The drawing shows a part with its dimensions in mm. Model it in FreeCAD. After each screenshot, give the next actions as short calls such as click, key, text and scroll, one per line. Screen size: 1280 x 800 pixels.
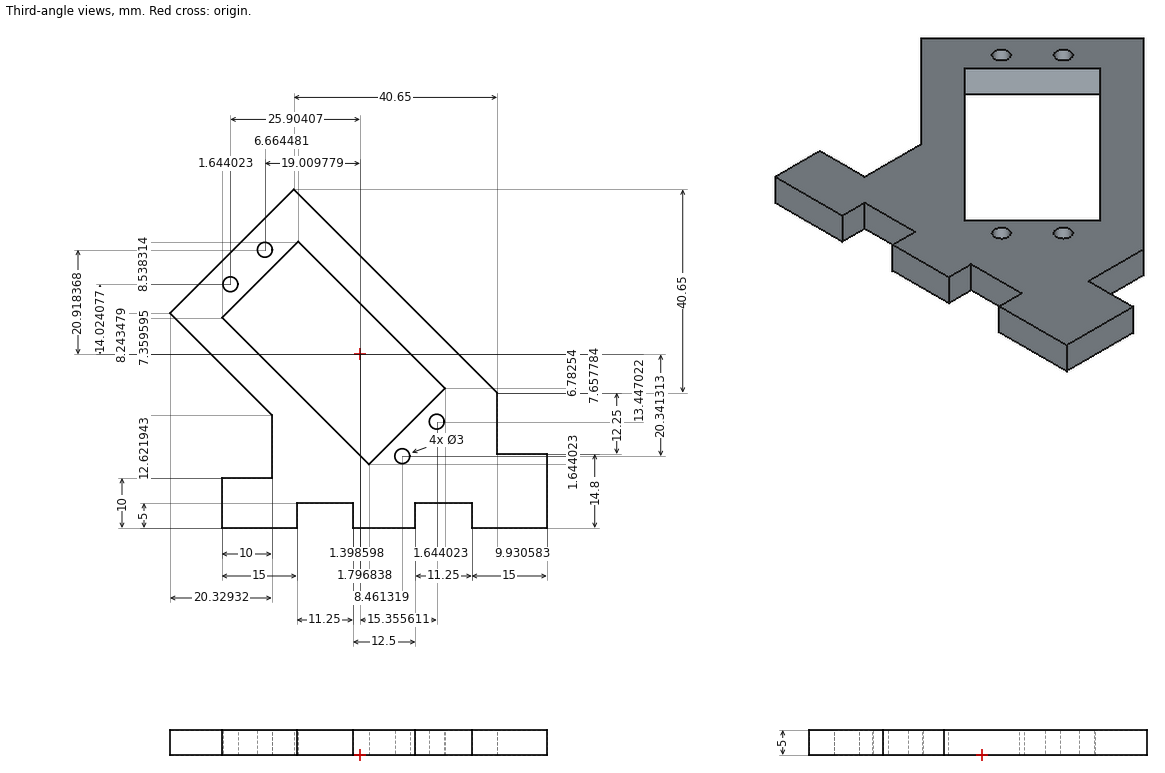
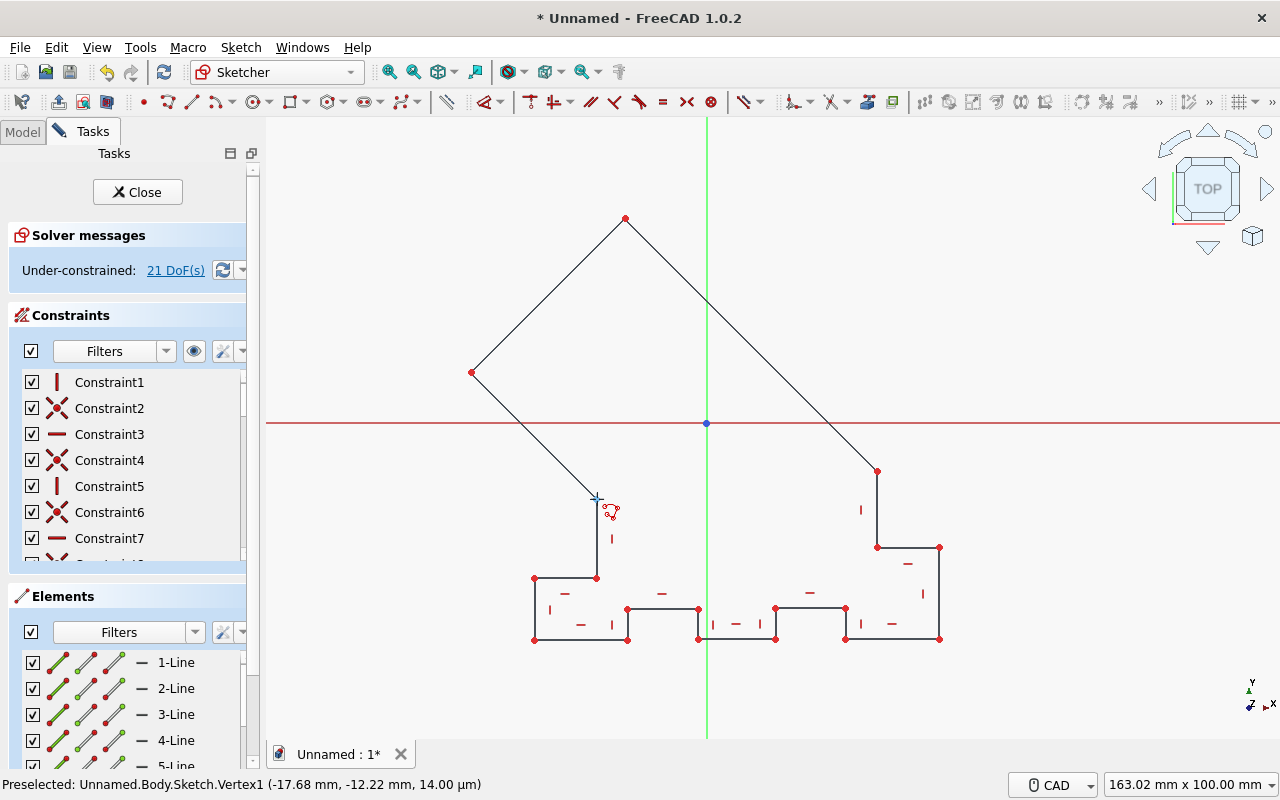
click(813, 465)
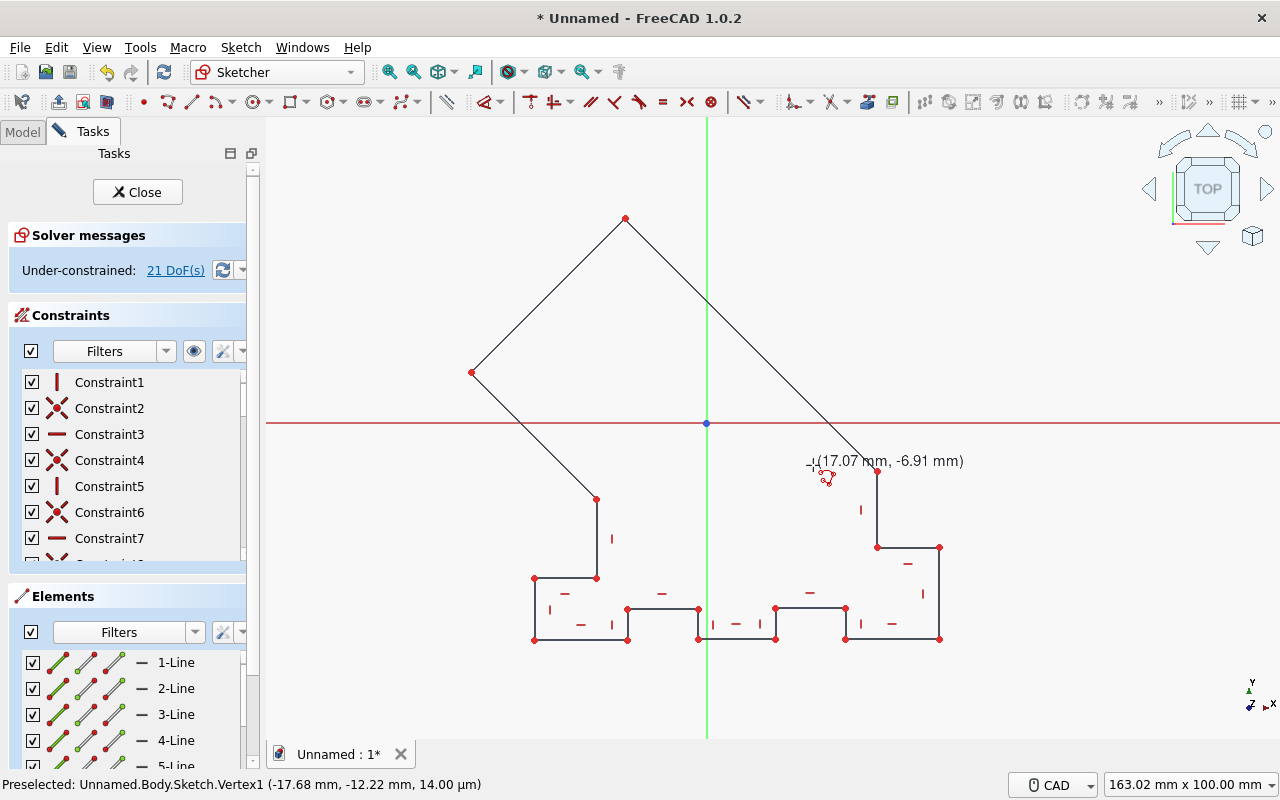
scroll(718, 560, up, 2)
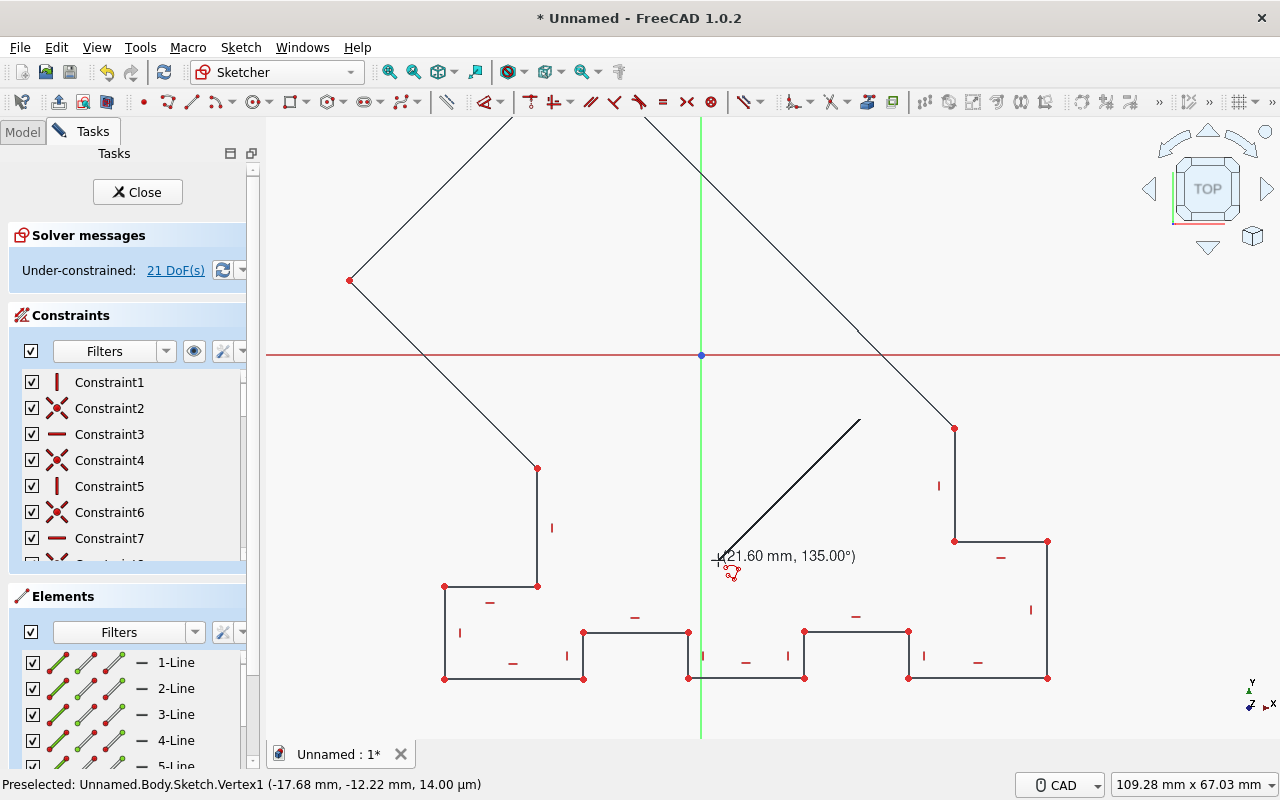
click(718, 559)
click(446, 287)
click(587, 146)
click(860, 419)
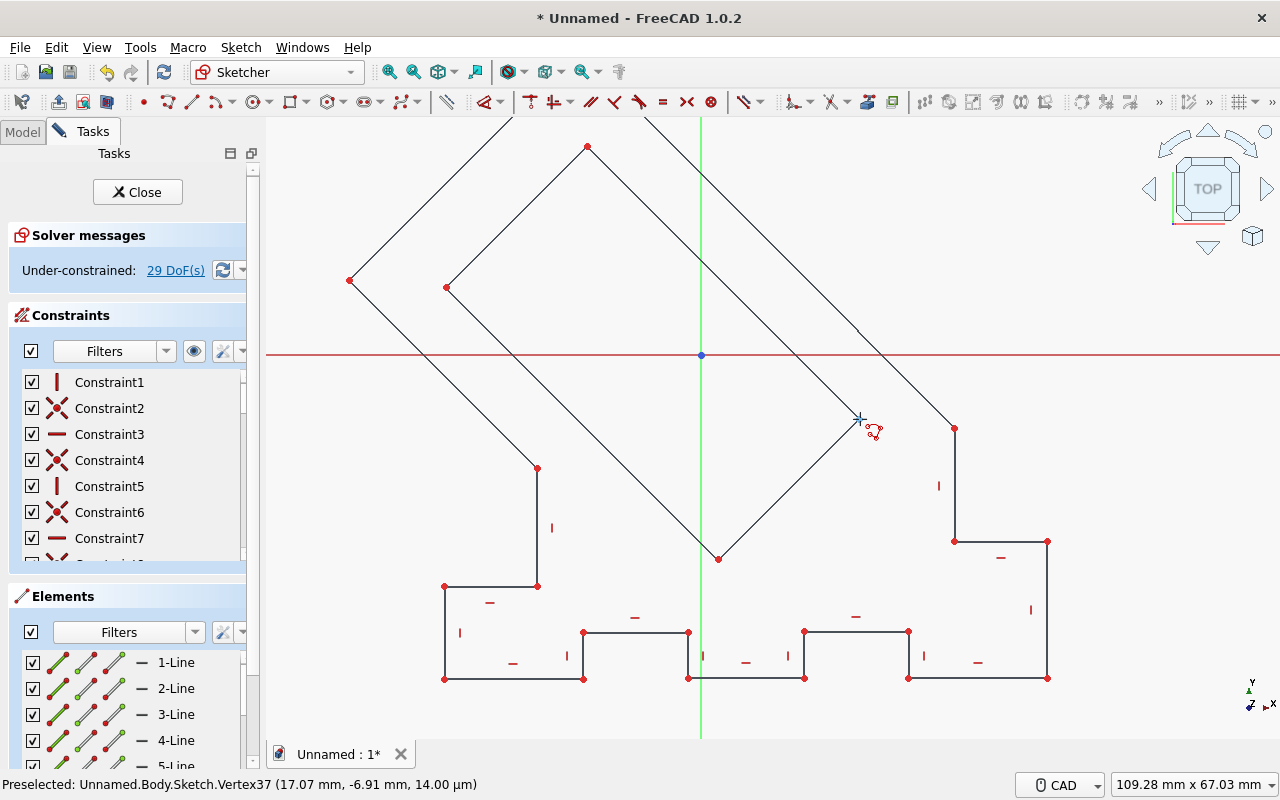
key(g)
key(c)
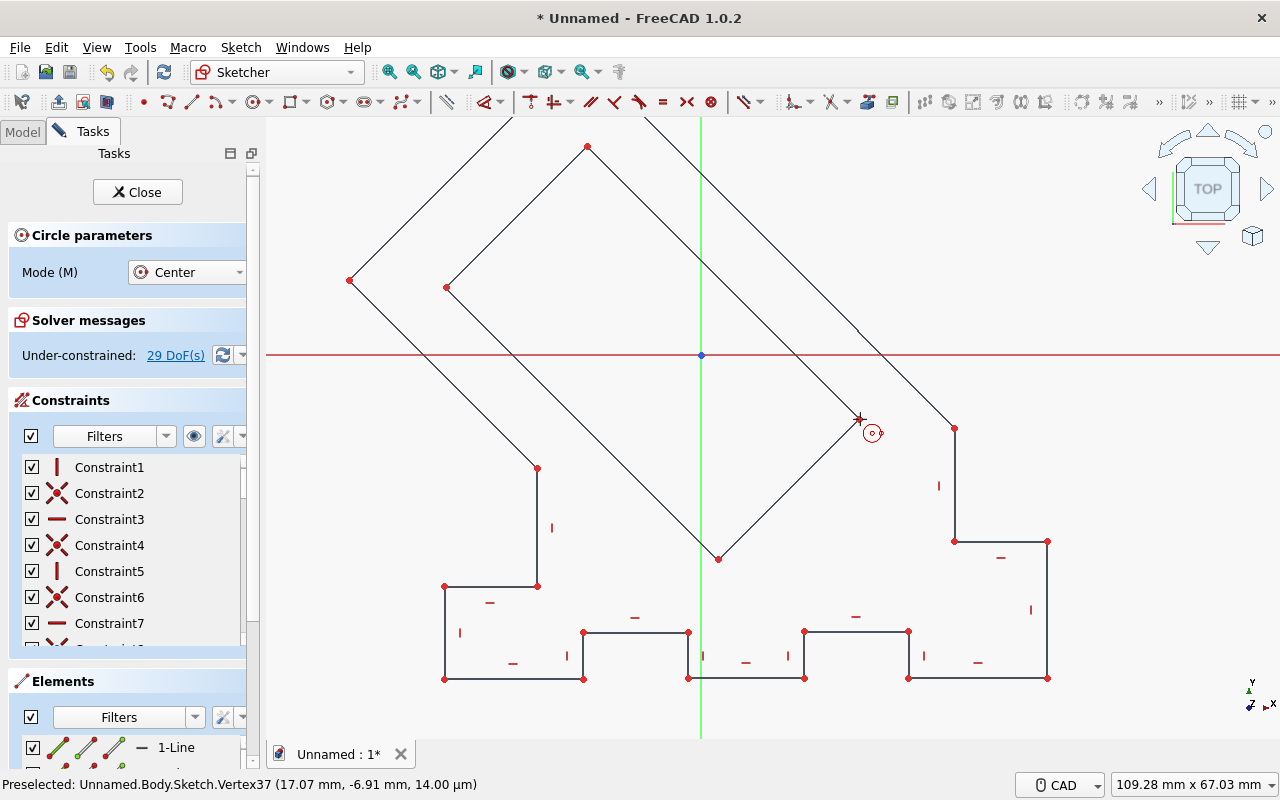
scroll(780, 544, up, 3)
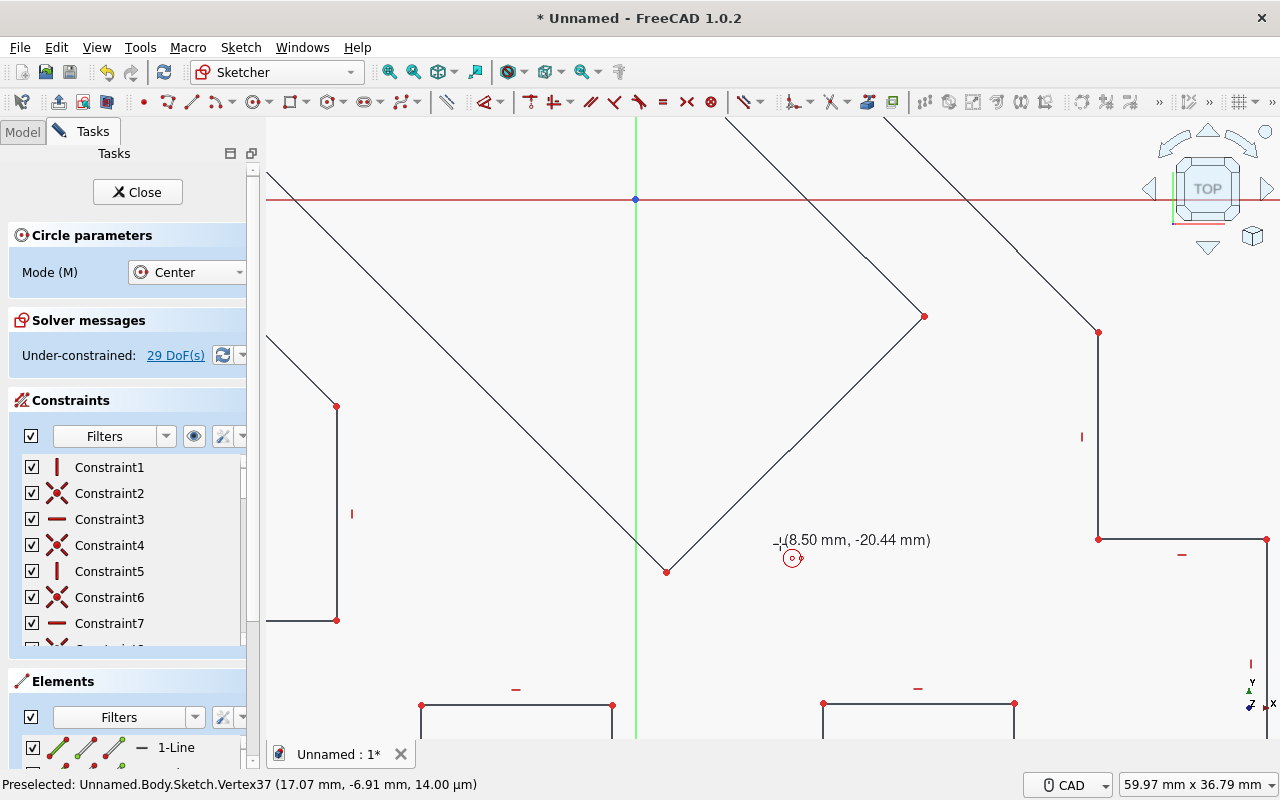
click(779, 544)
click(797, 526)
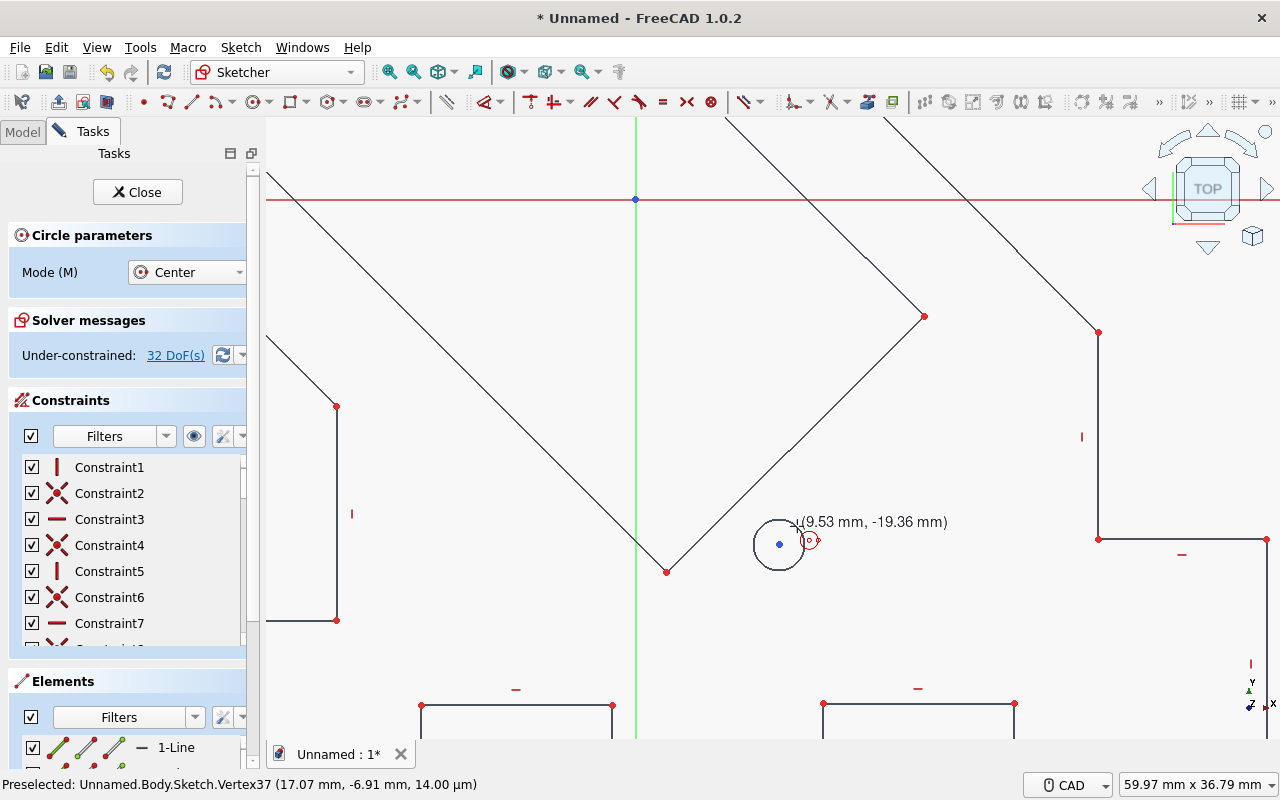
click(896, 427)
click(913, 409)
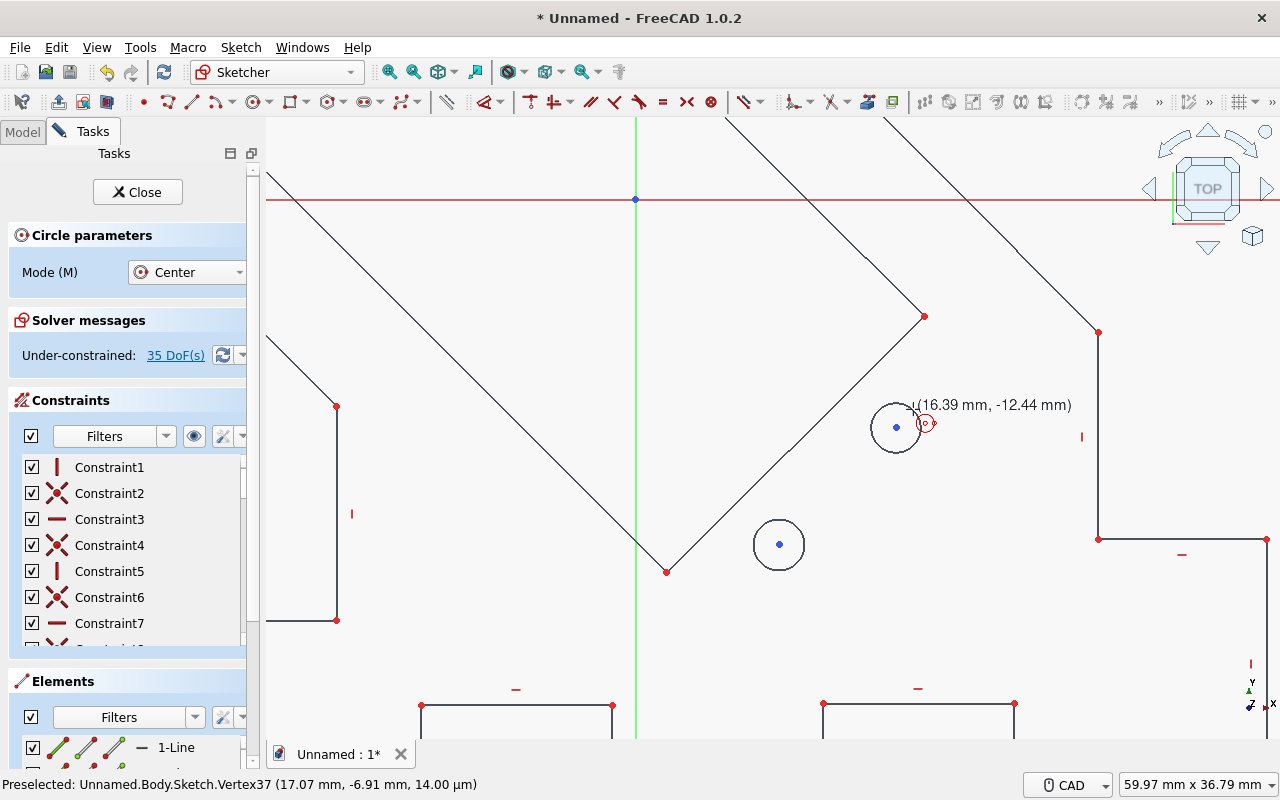
scroll(747, 552, down, 5)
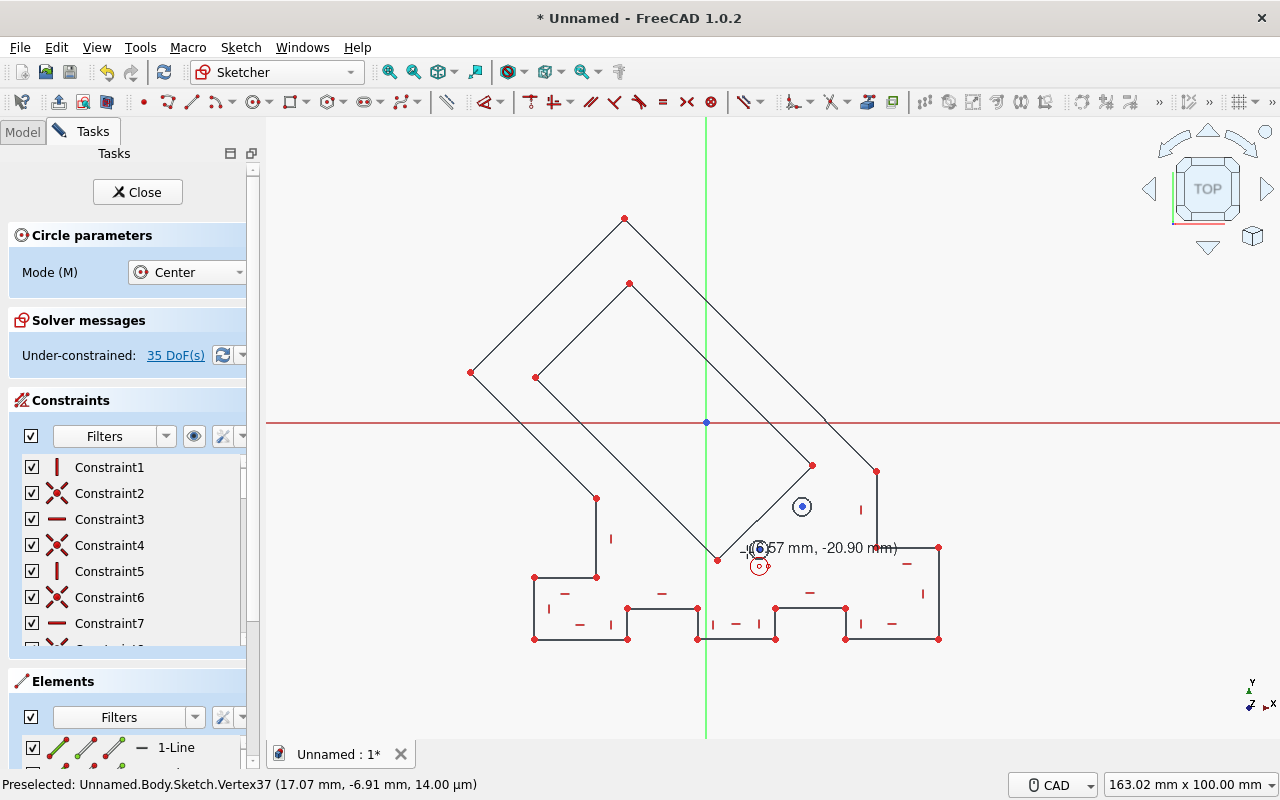
scroll(545, 336, up, 5)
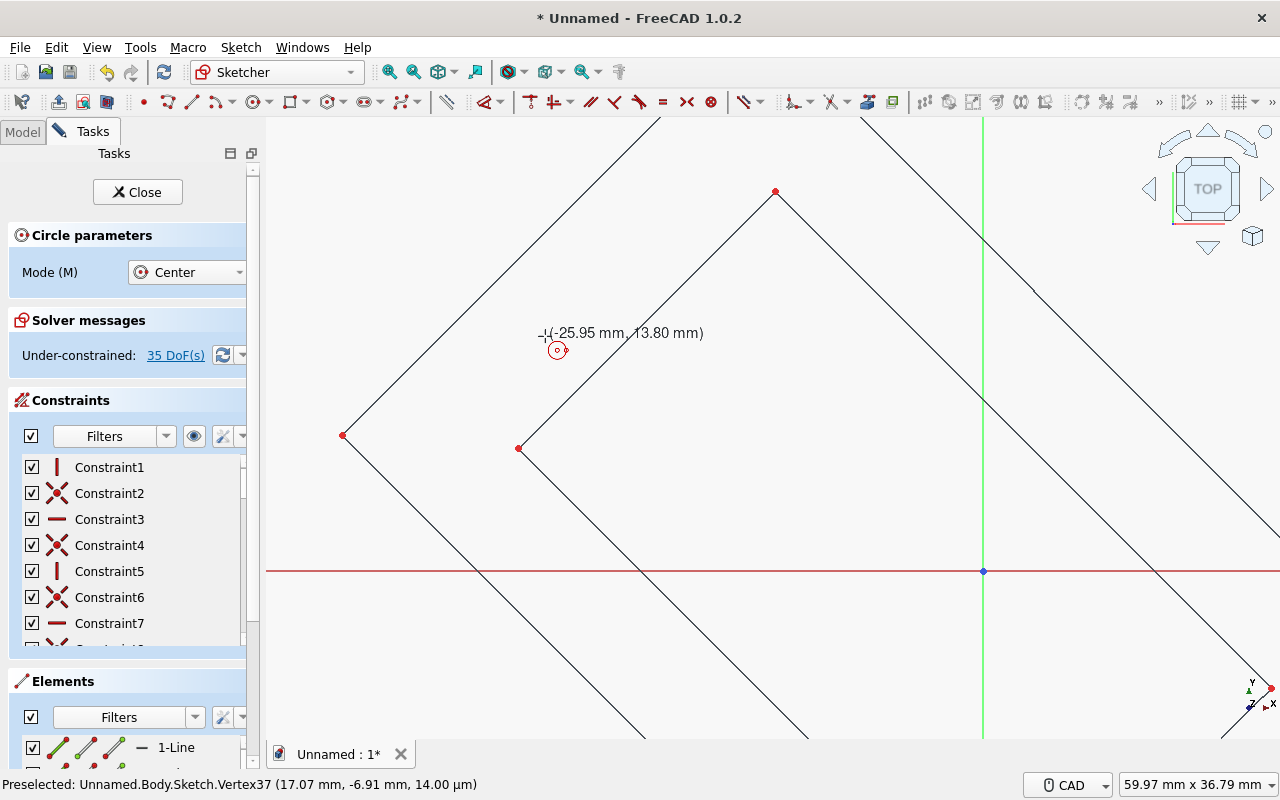
click(545, 334)
click(563, 316)